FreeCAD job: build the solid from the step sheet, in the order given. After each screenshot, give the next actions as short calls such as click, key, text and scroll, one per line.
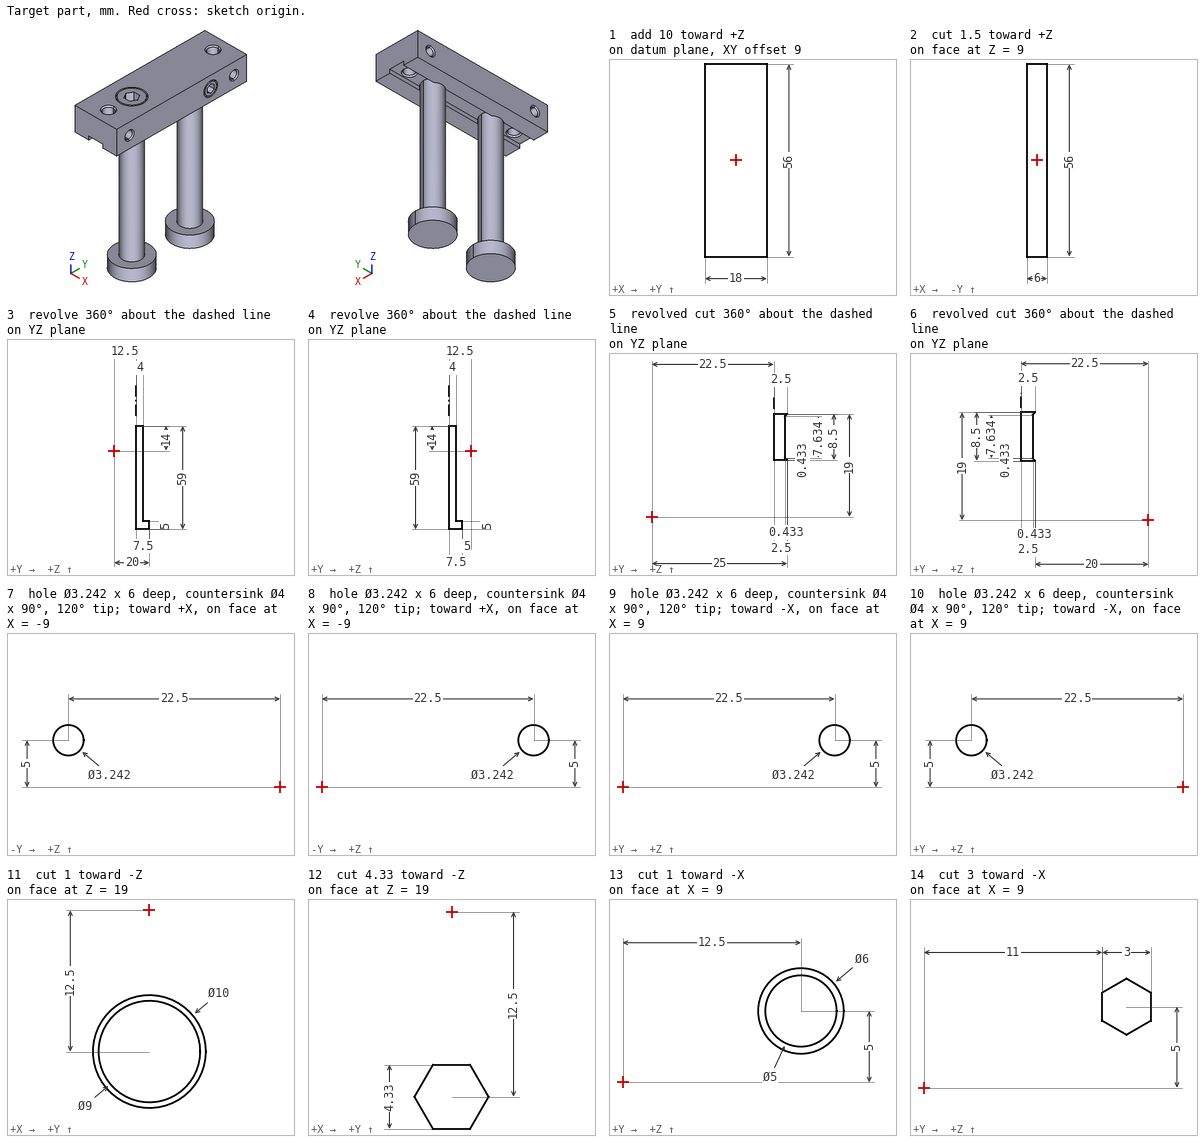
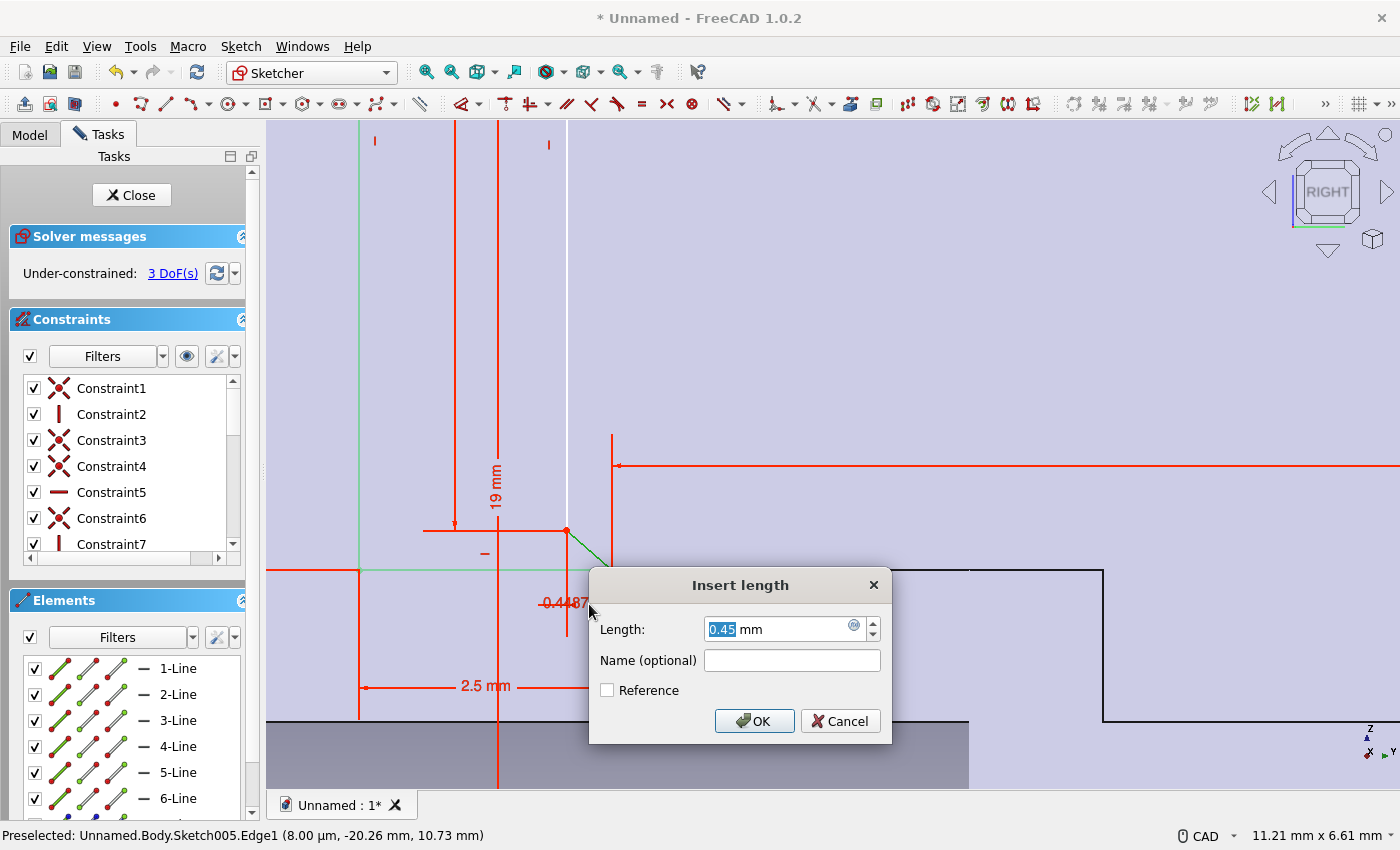
text(0.433)
key(Return)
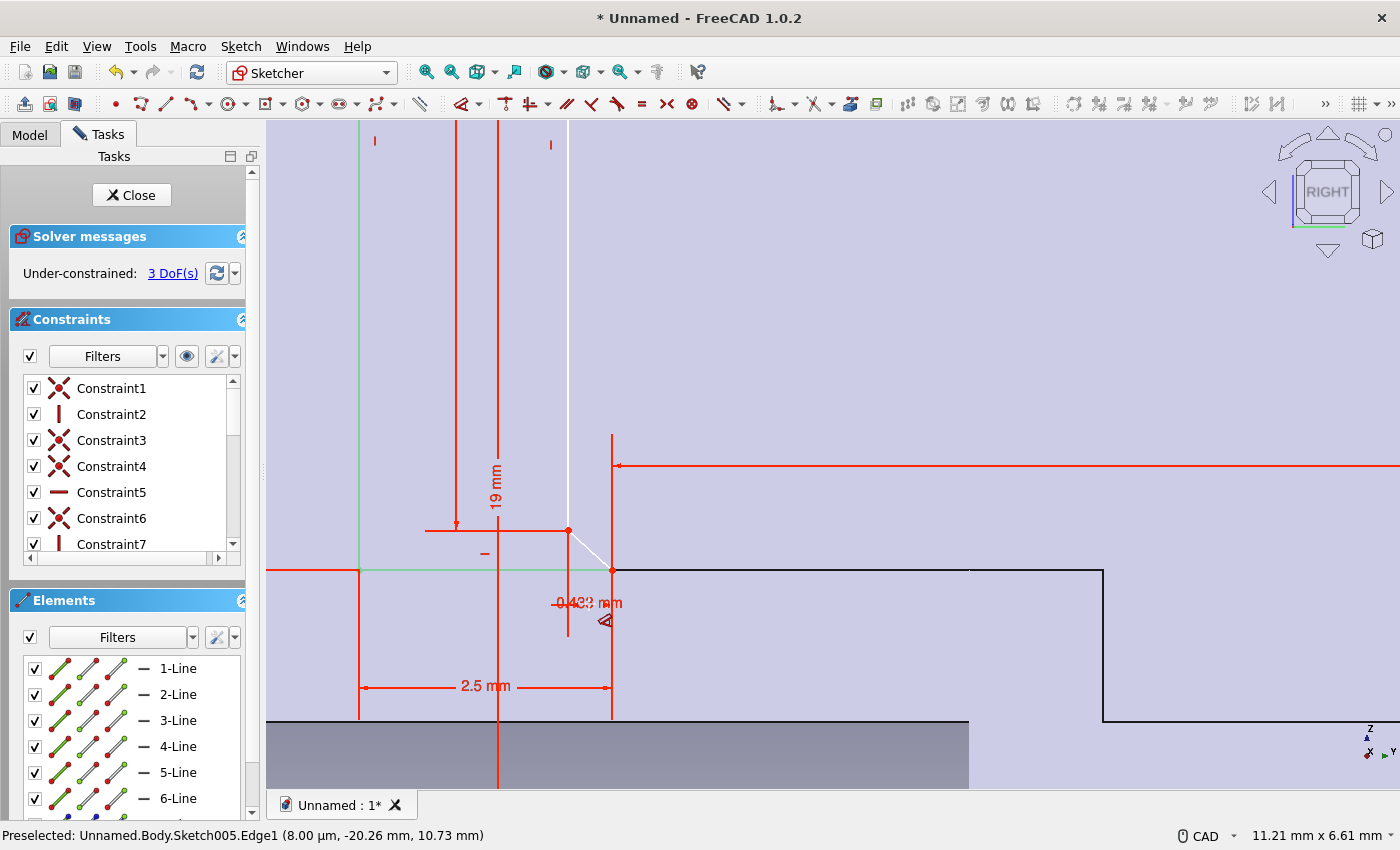
click(599, 558)
click(534, 551)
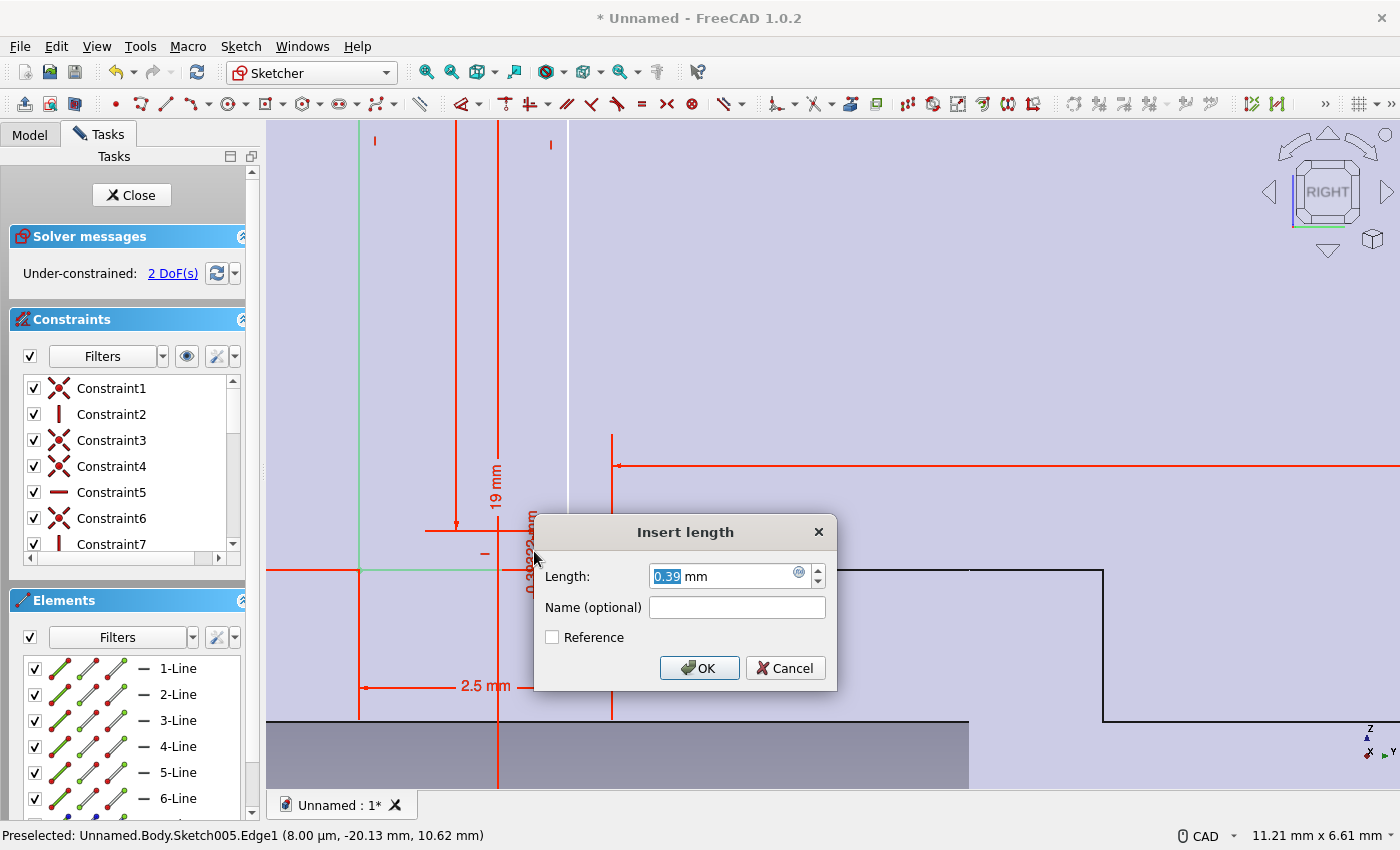
text(0.433)
key(Return)
key(Escape)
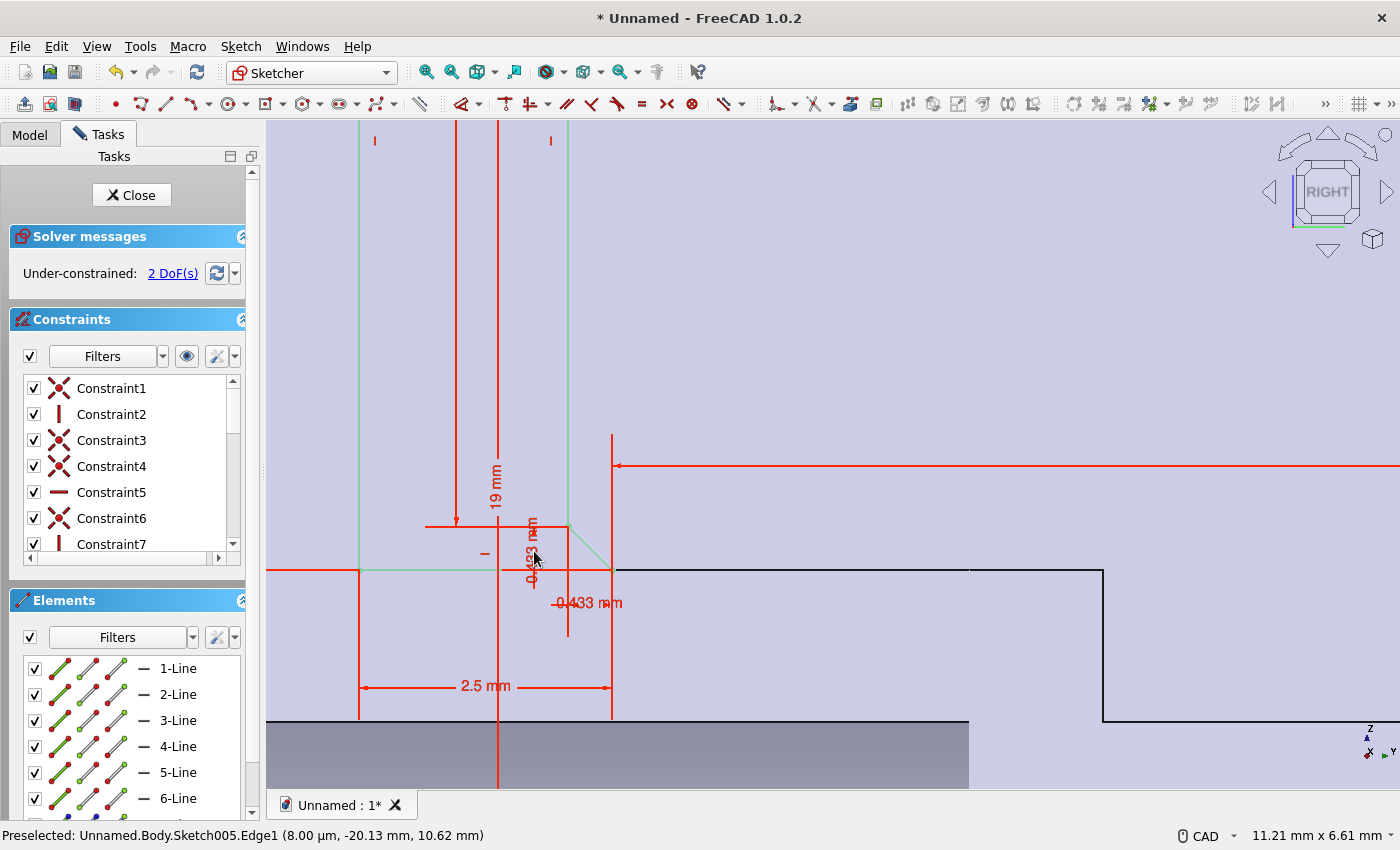
click(132, 195)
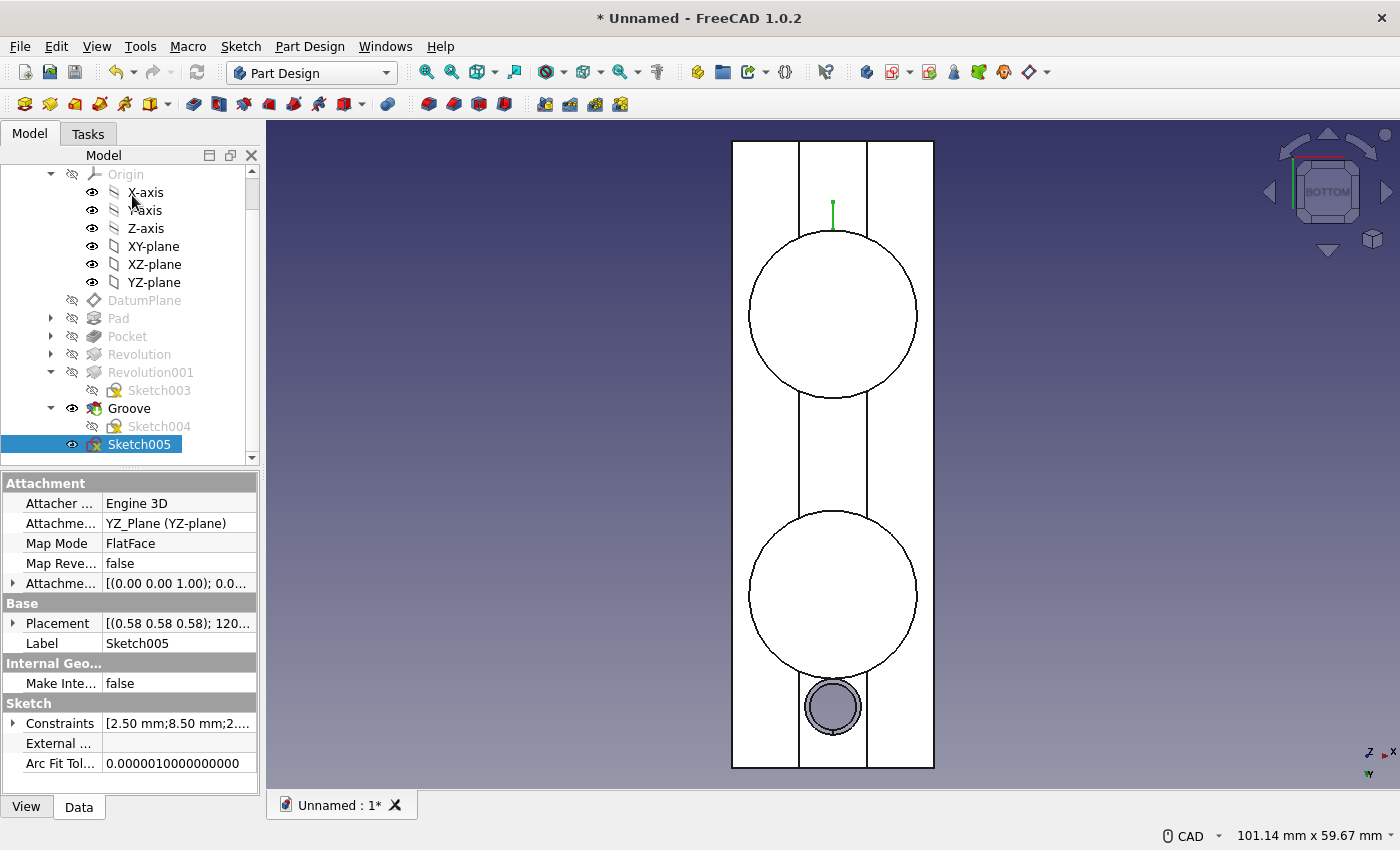
click(244, 104)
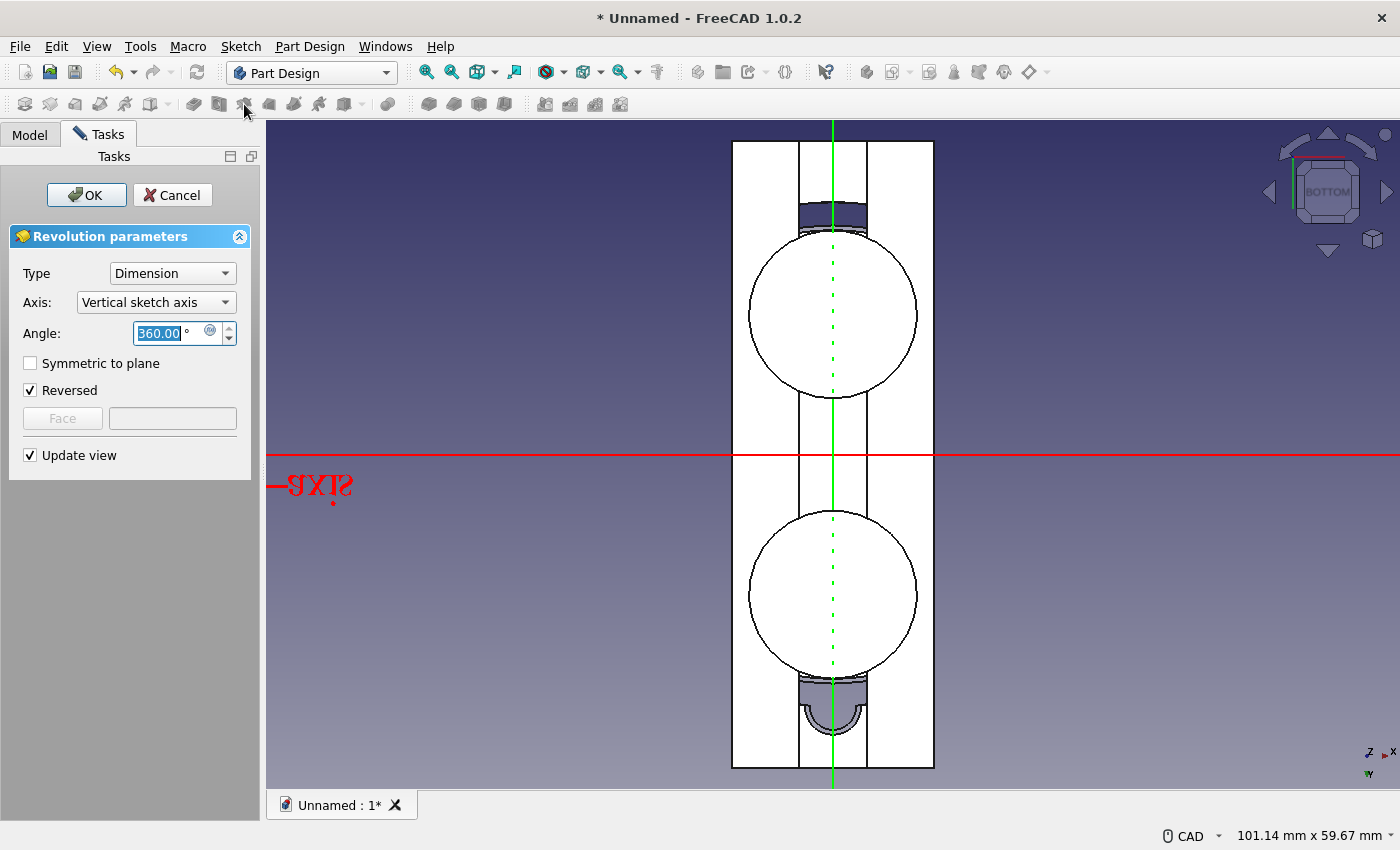
click(157, 302)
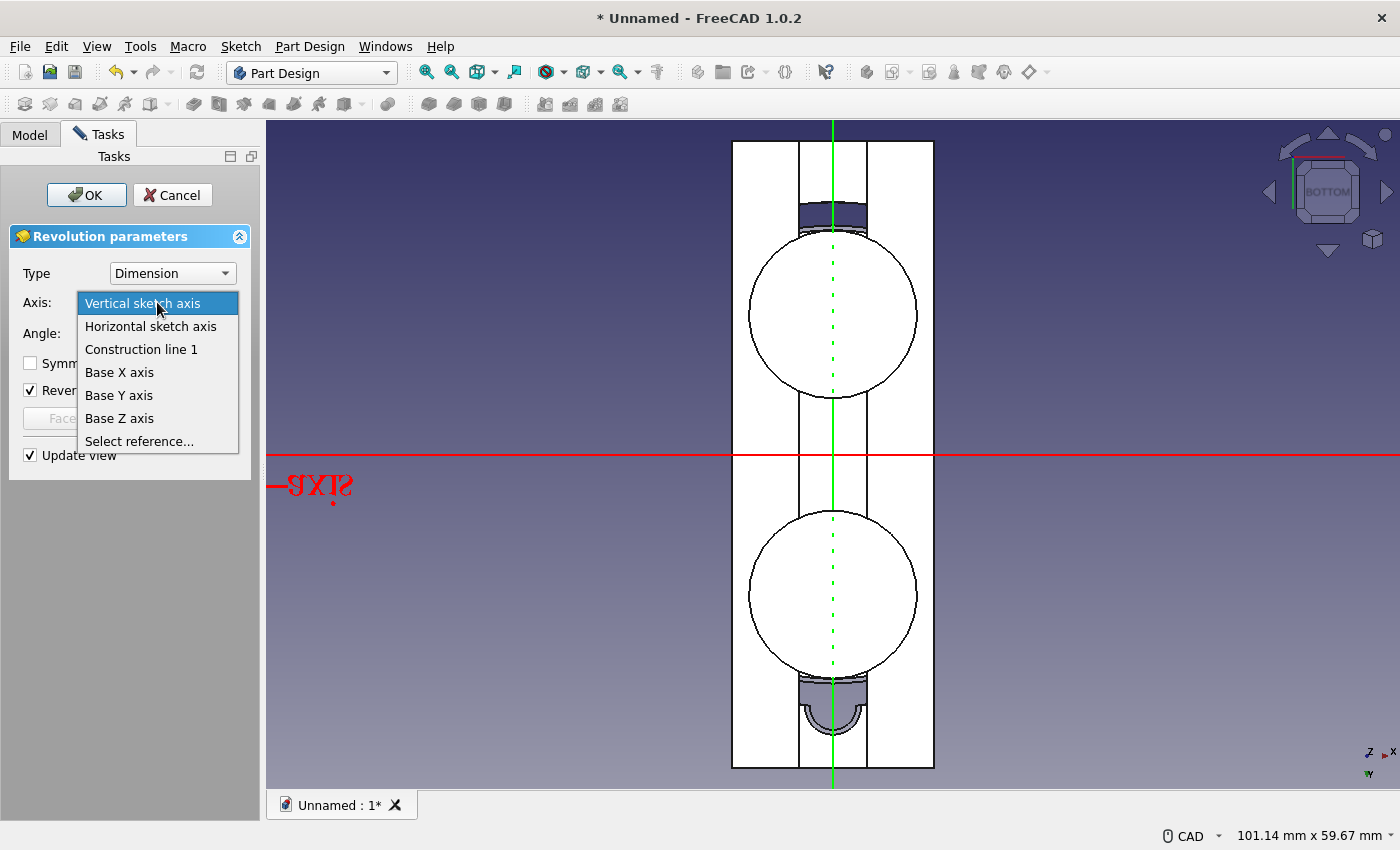
click(156, 350)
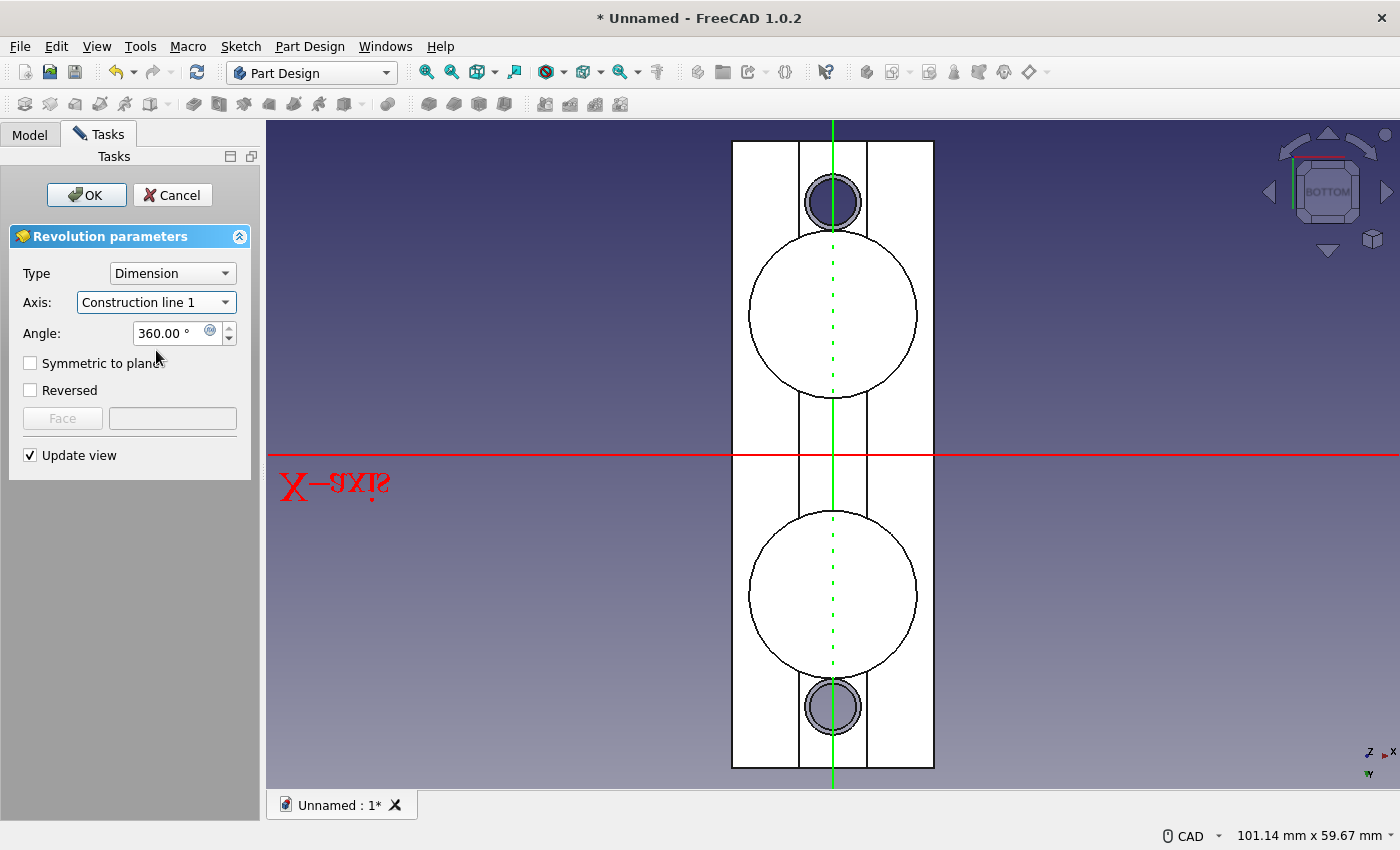
click(87, 195)